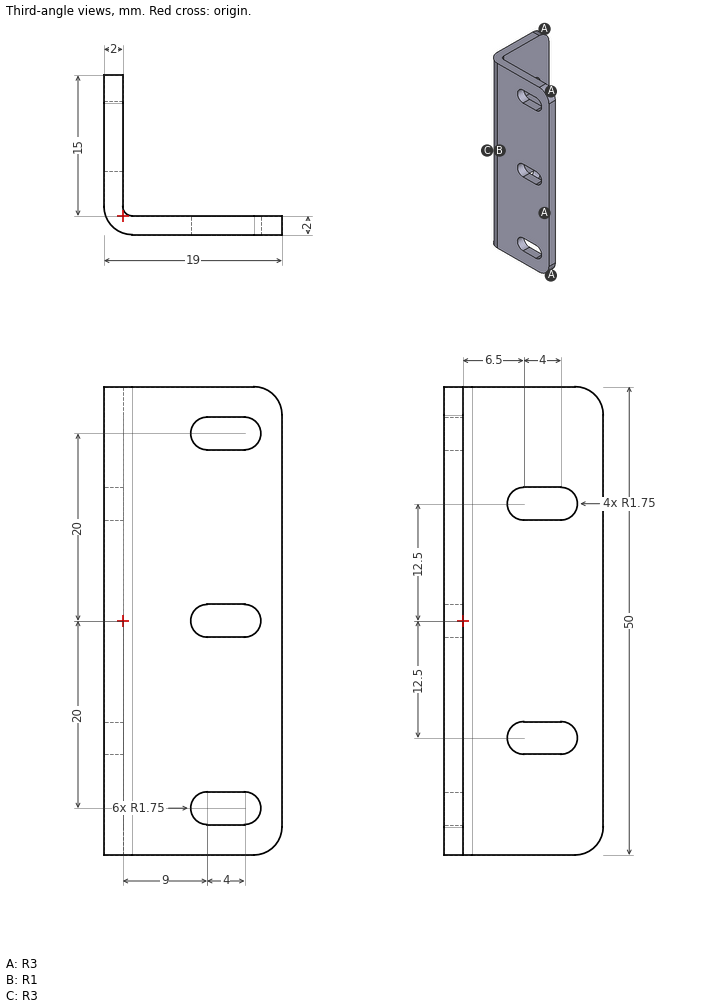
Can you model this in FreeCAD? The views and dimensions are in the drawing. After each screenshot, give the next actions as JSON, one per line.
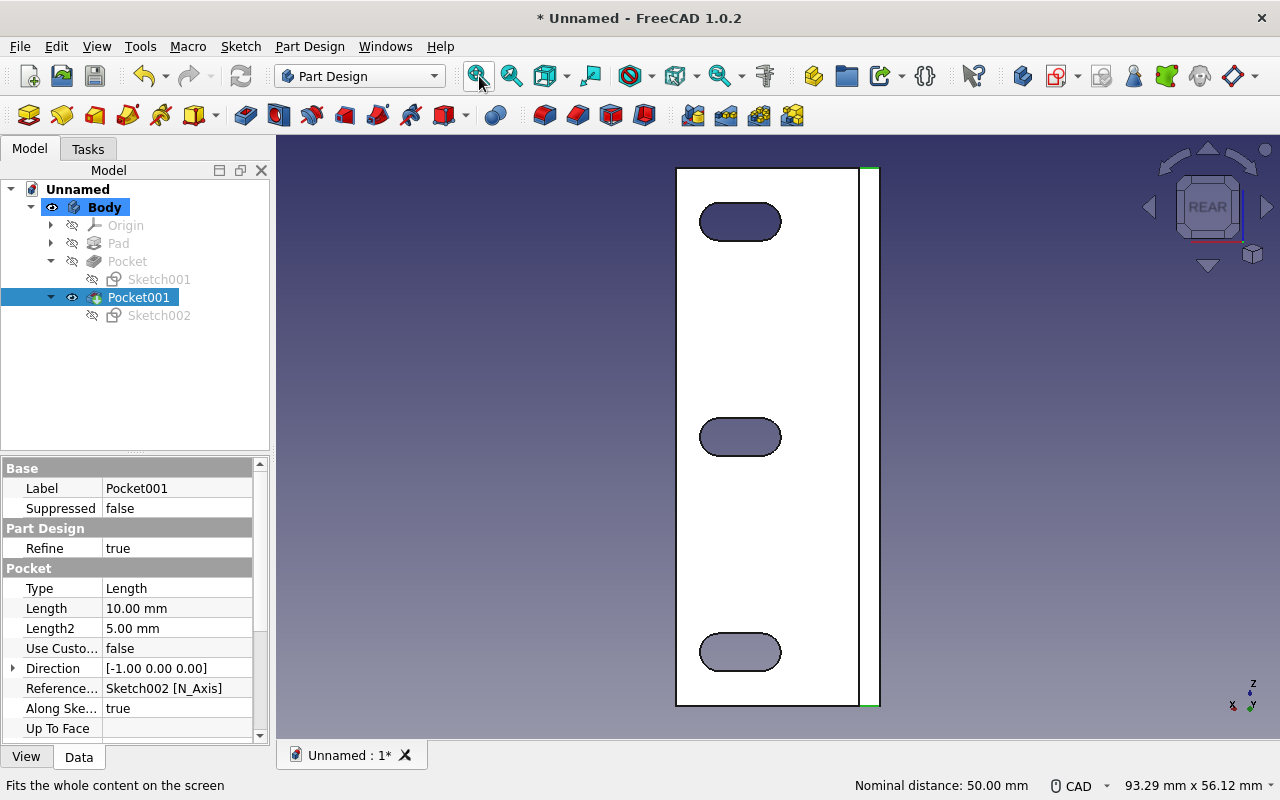
{"action": "key", "text": "0"}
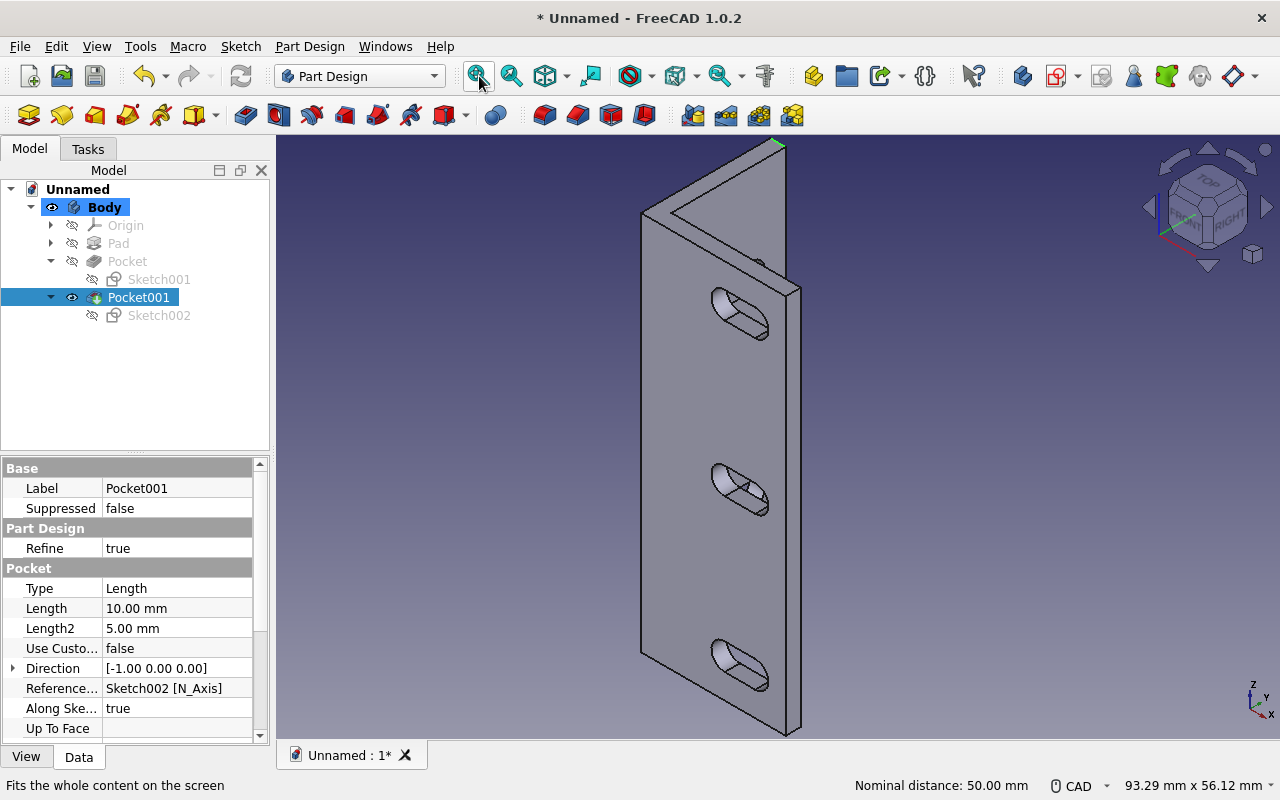
{"action": "left_click", "coordinate": [793, 291], "text": "ctrl"}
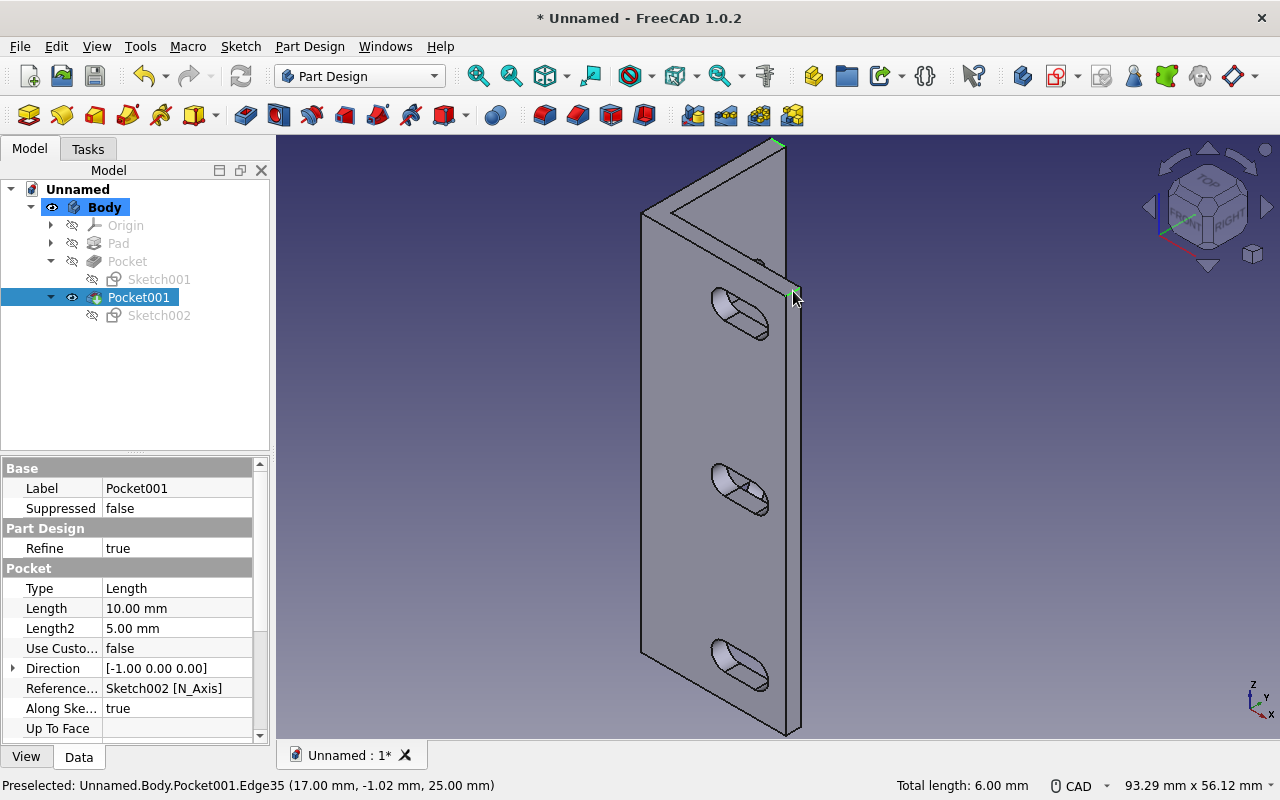
{"action": "key", "text": "2"}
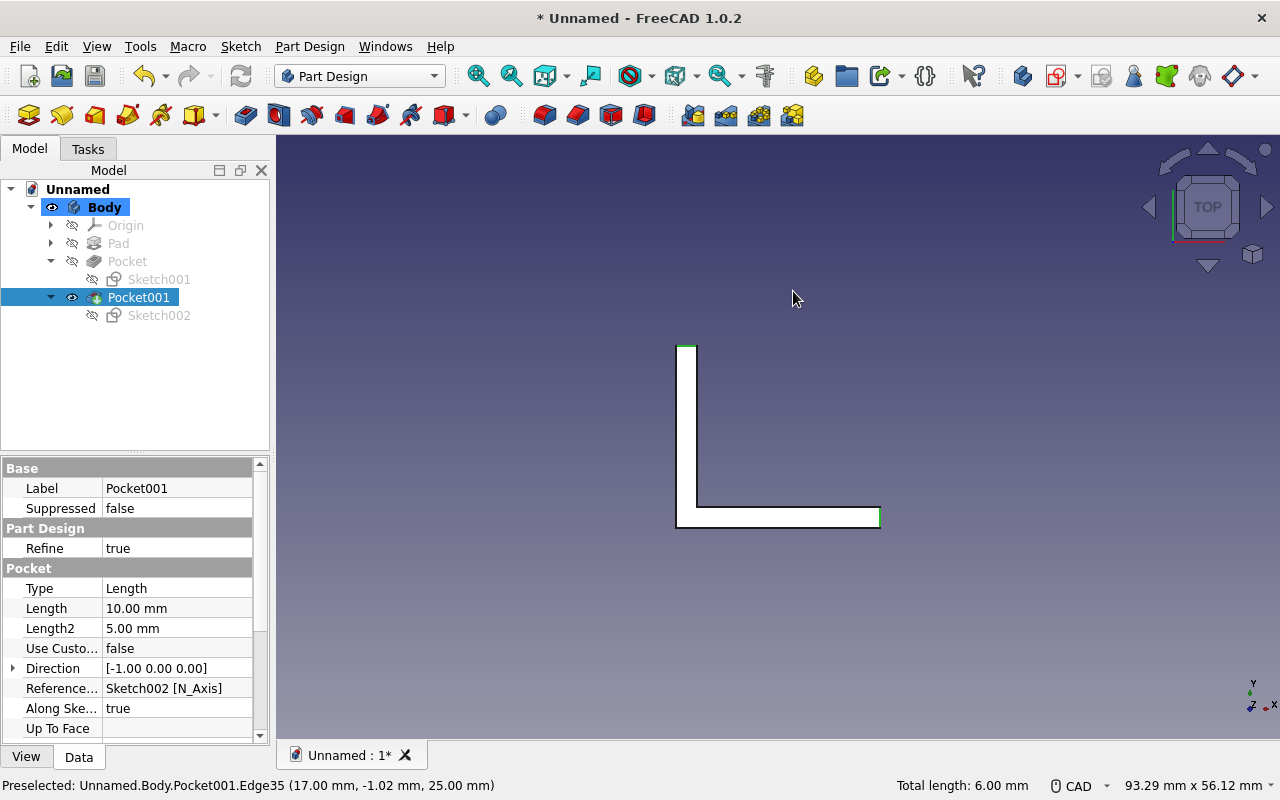
{"action": "left_click", "coordinate": [479, 76]}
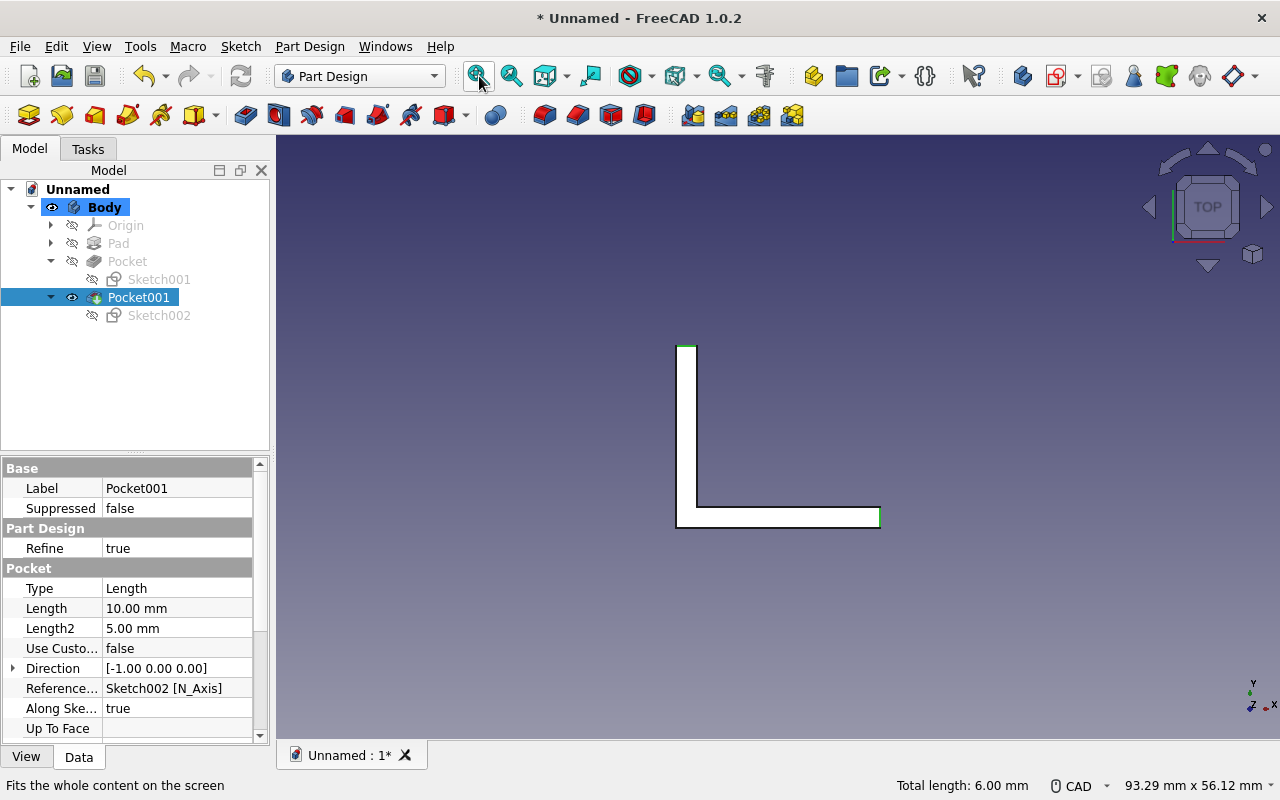
{"action": "scroll", "coordinate": [880, 517], "scroll_direction": "up", "scroll_amount": 4}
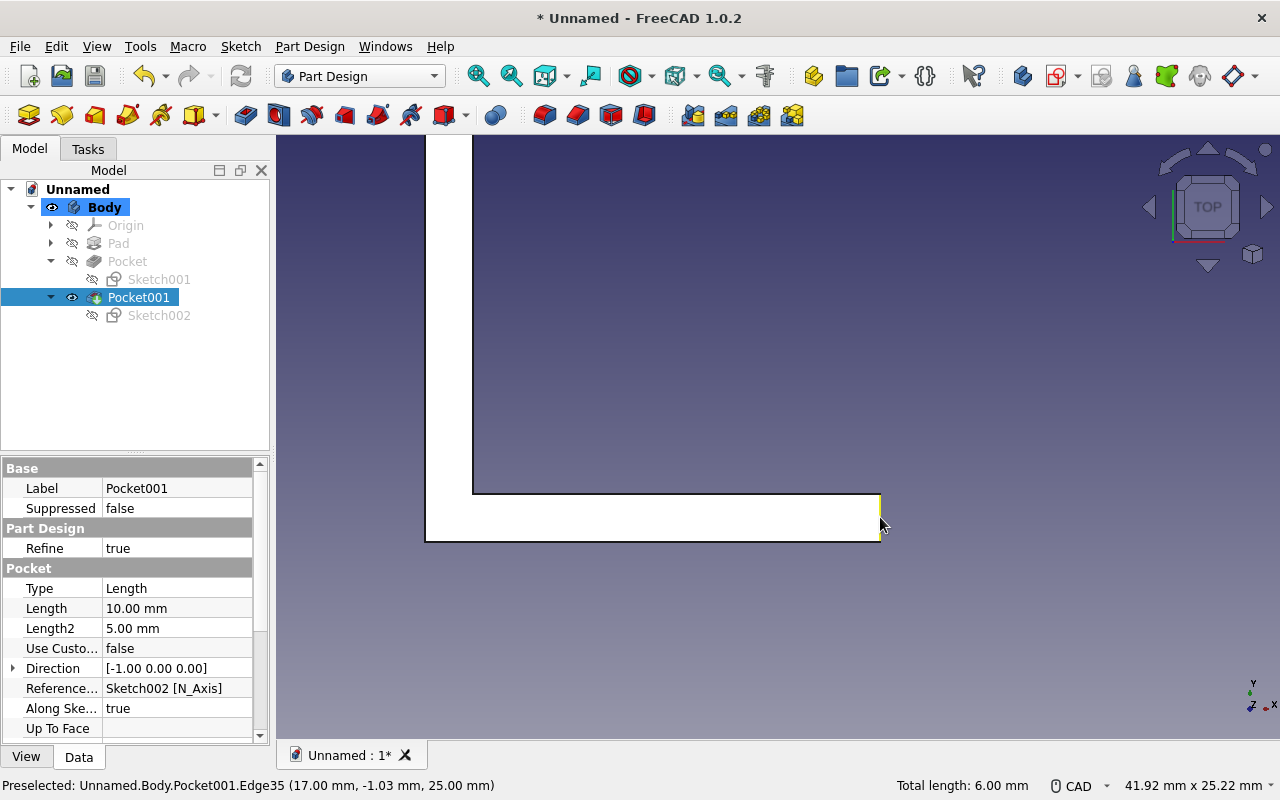
{"action": "left_click", "coordinate": [479, 76]}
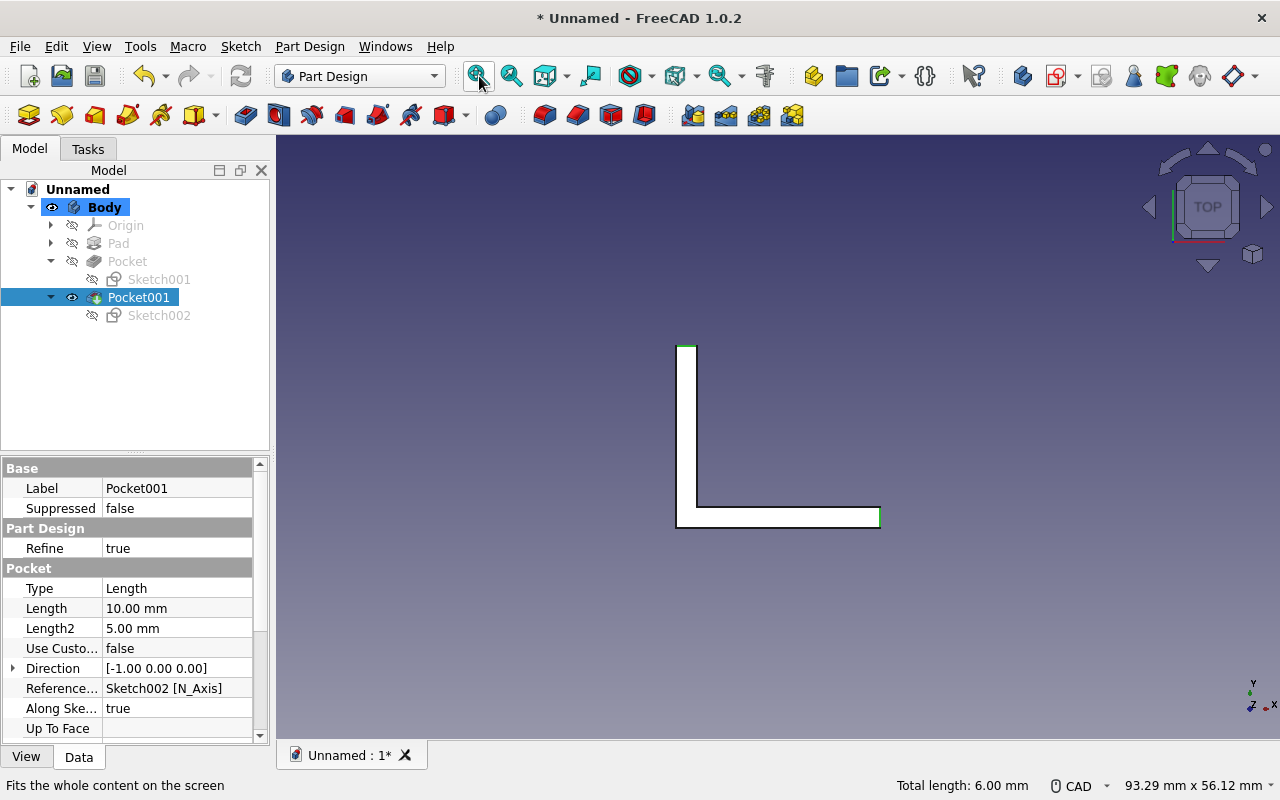
{"action": "key", "text": "1"}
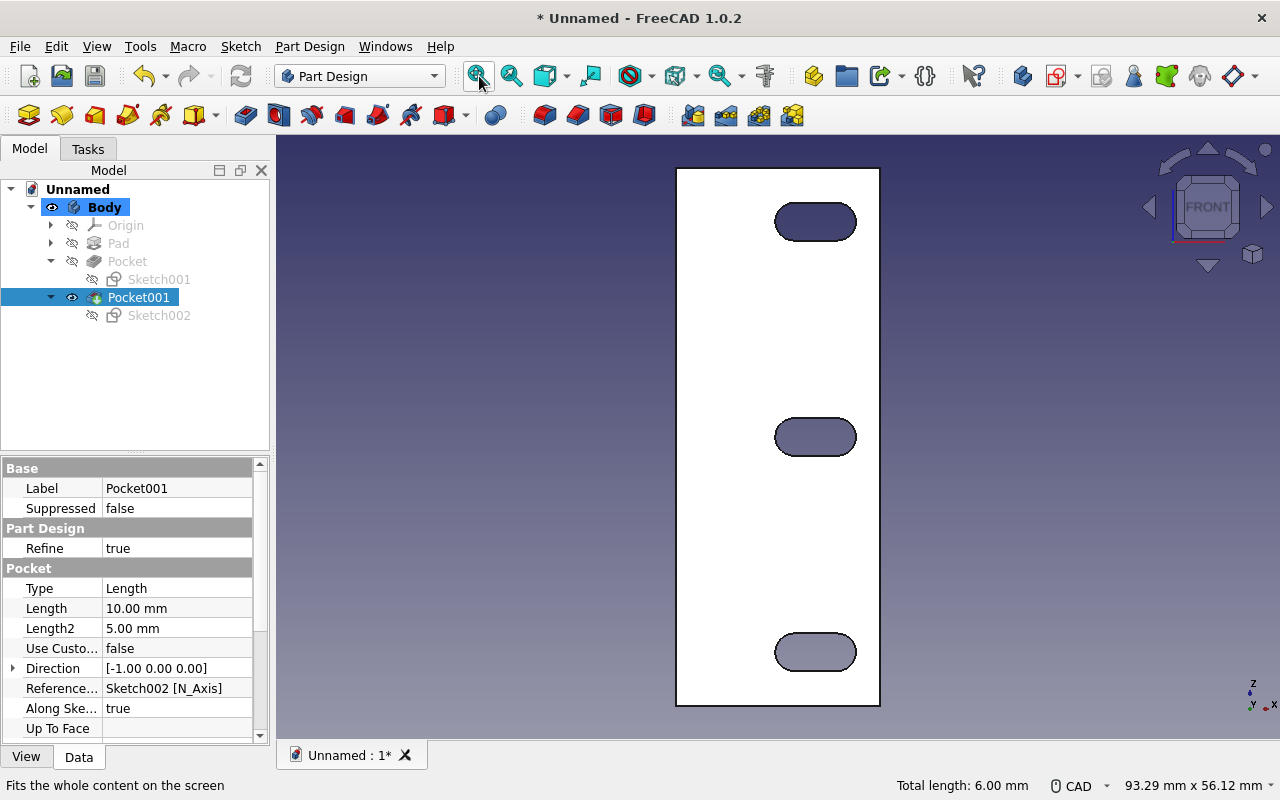
{"action": "scroll", "coordinate": [880, 705], "scroll_direction": "up", "scroll_amount": 4}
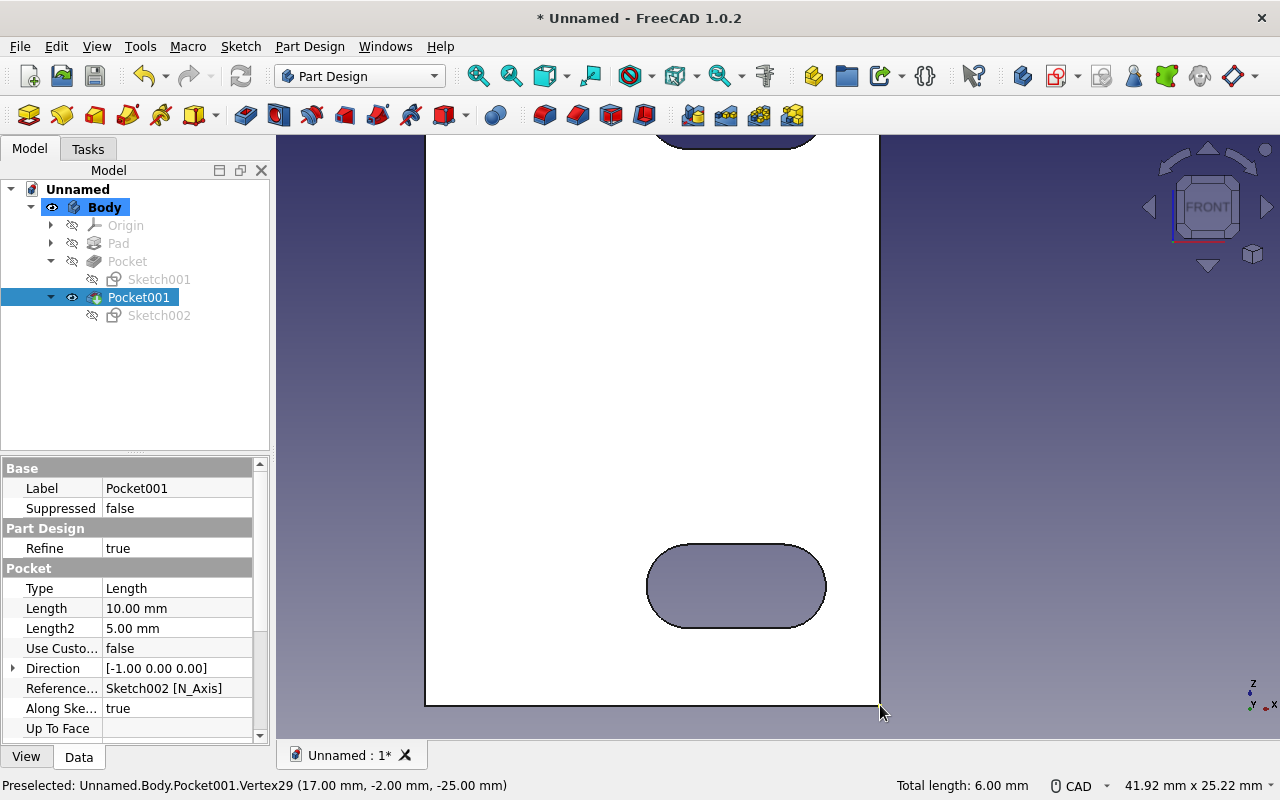
{"action": "left_click", "coordinate": [479, 76]}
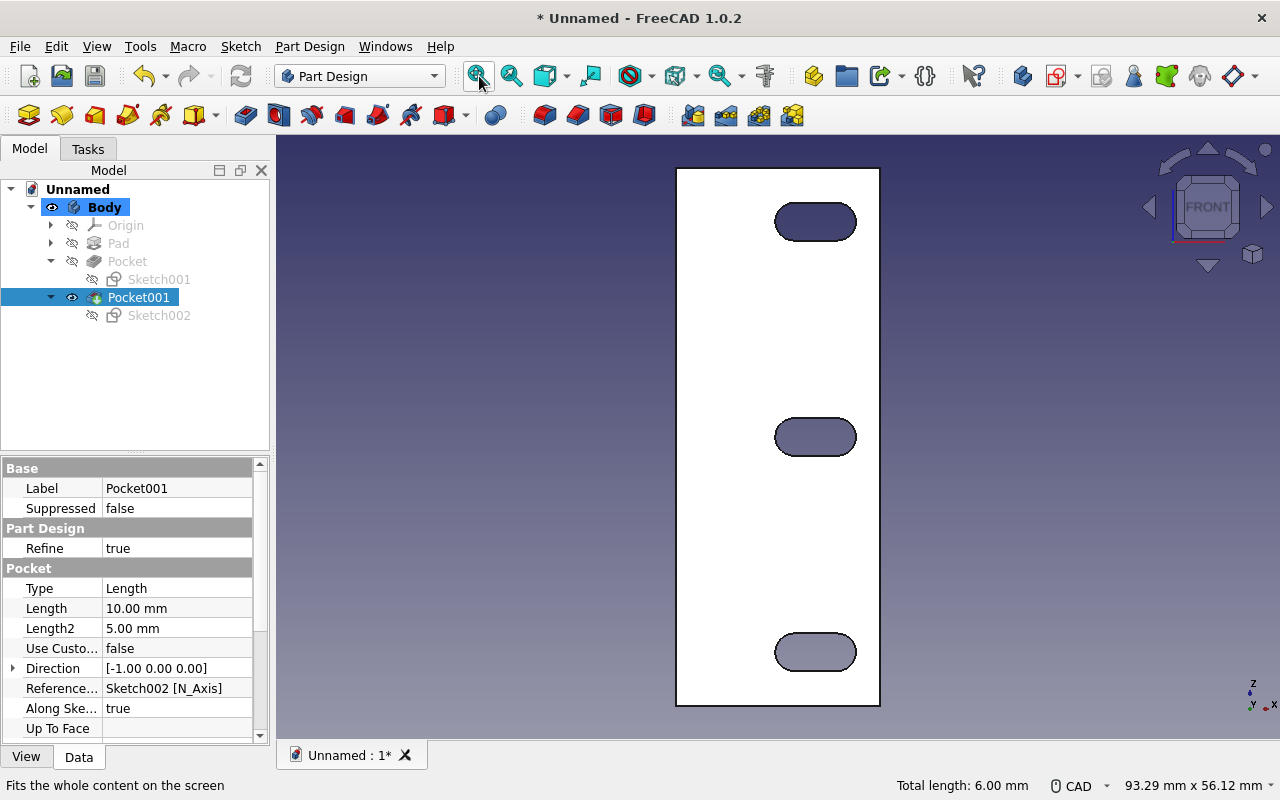
{"action": "key", "text": "3"}